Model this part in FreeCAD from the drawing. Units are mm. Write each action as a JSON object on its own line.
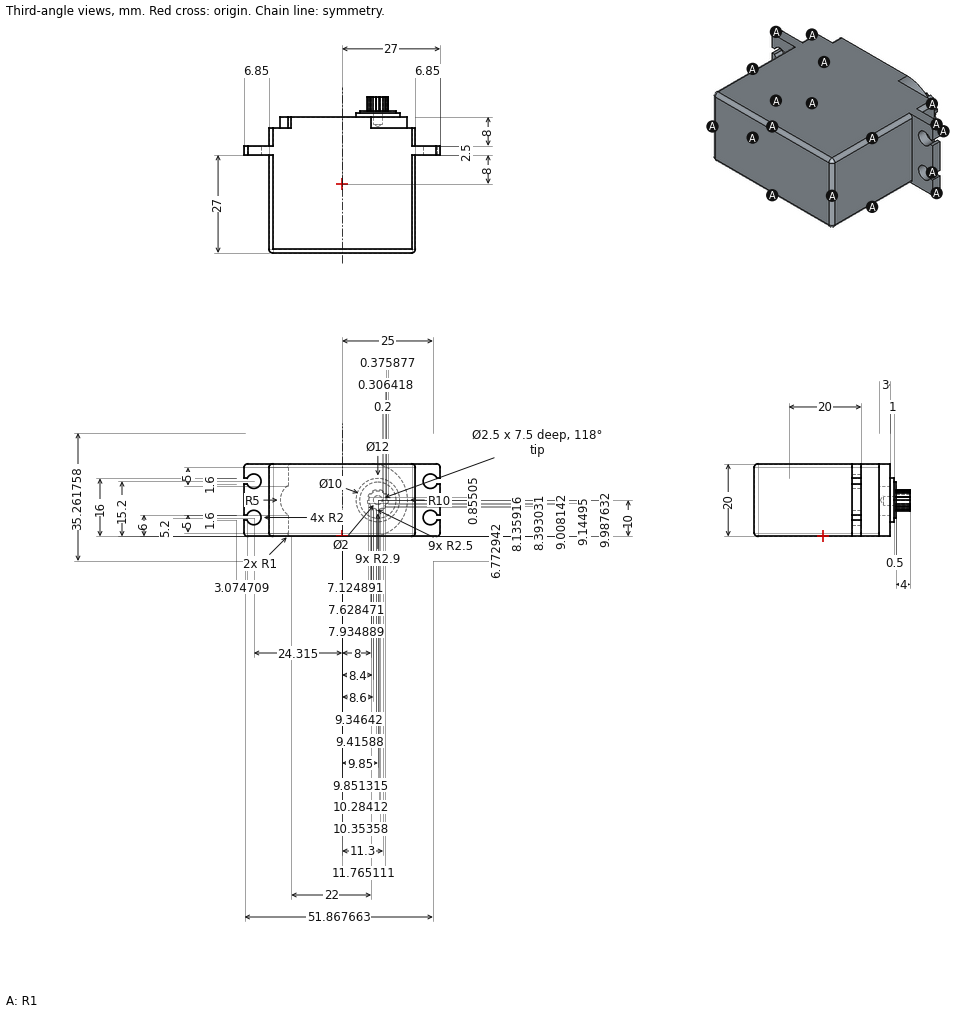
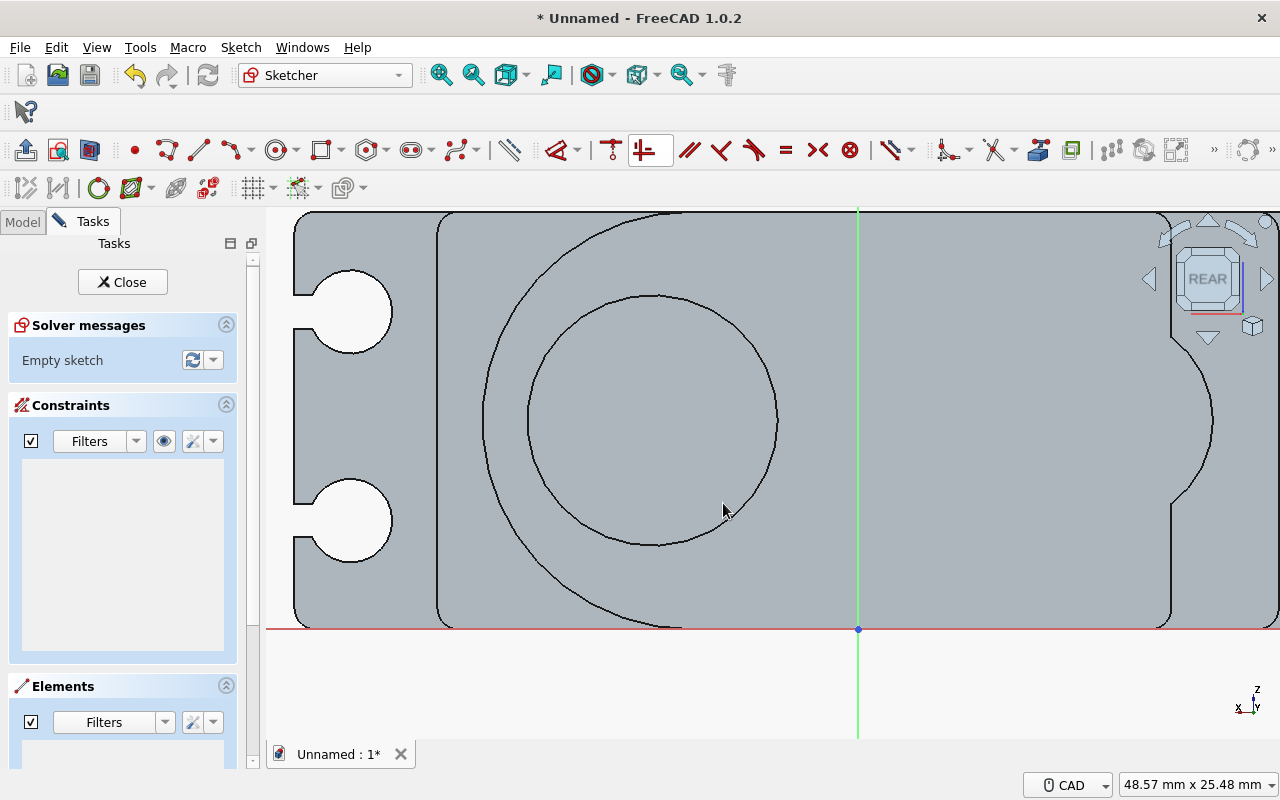
{"action": "left_click", "coordinate": [276, 150]}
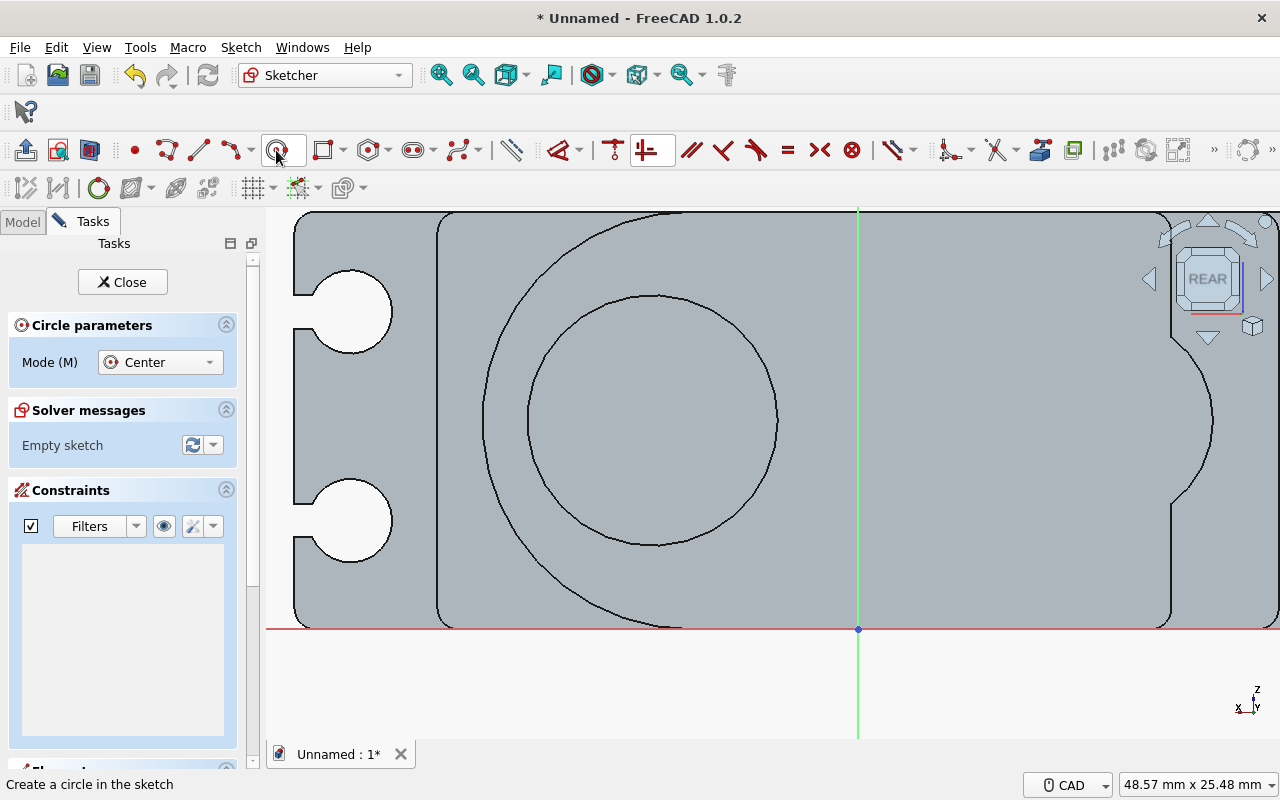
{"action": "left_click", "coordinate": [652, 421]}
{"action": "mouse_move", "coordinate": [726, 347]}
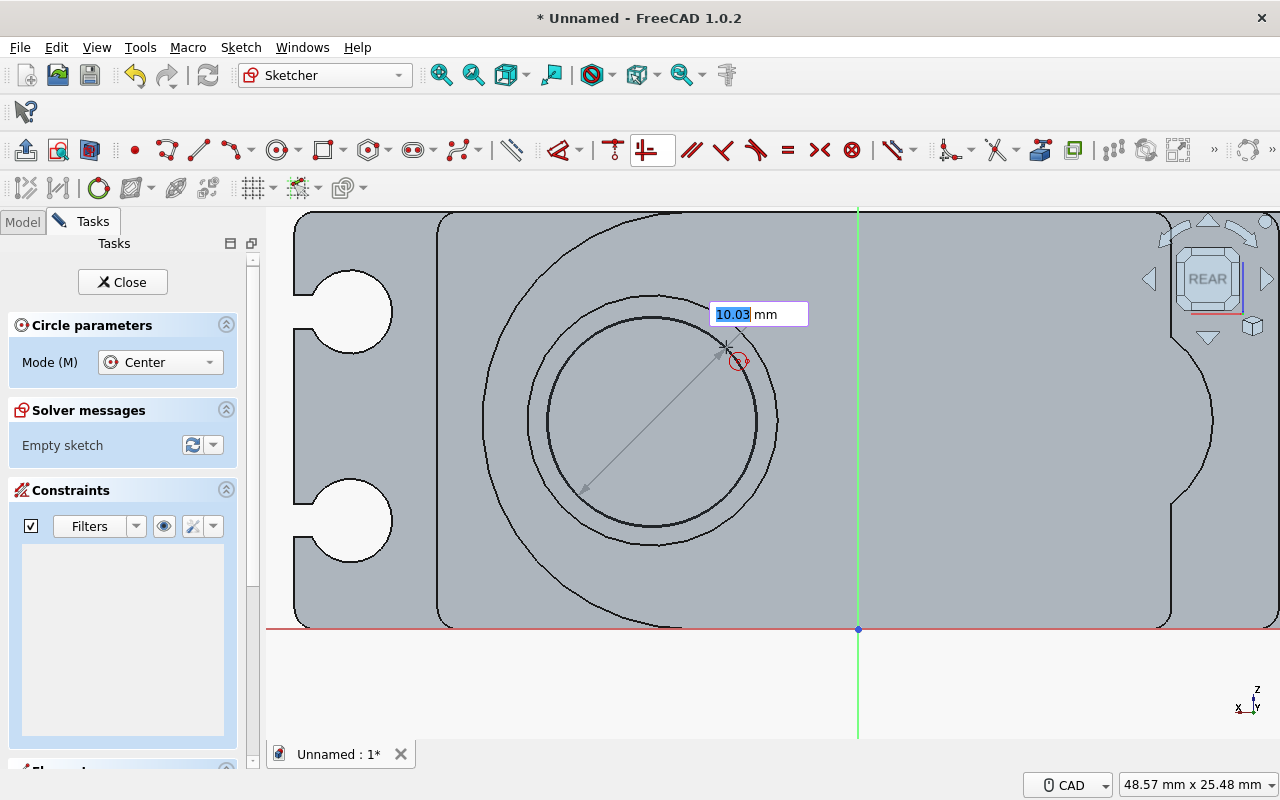
{"action": "type", "text": "10"}
{"action": "key", "text": "Return"}
{"action": "key", "text": "Escape"}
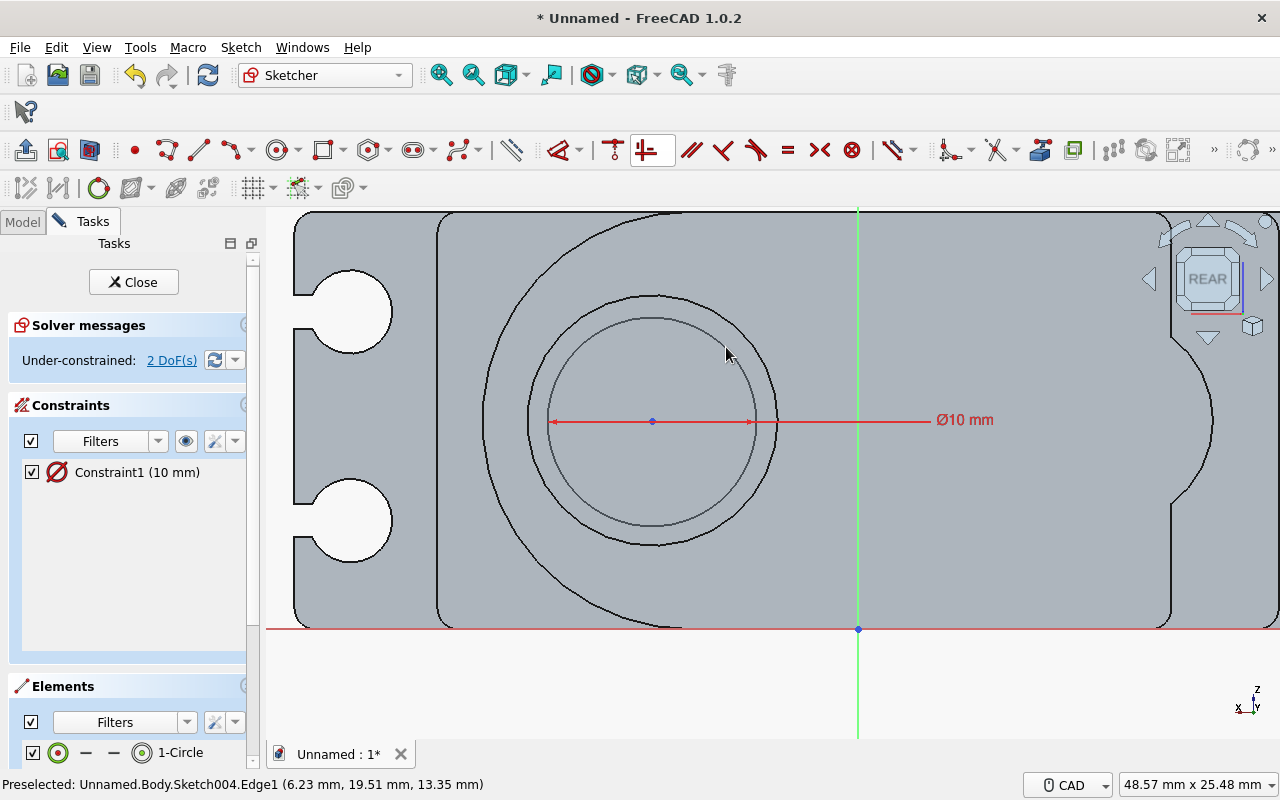
{"action": "left_click", "coordinate": [558, 150]}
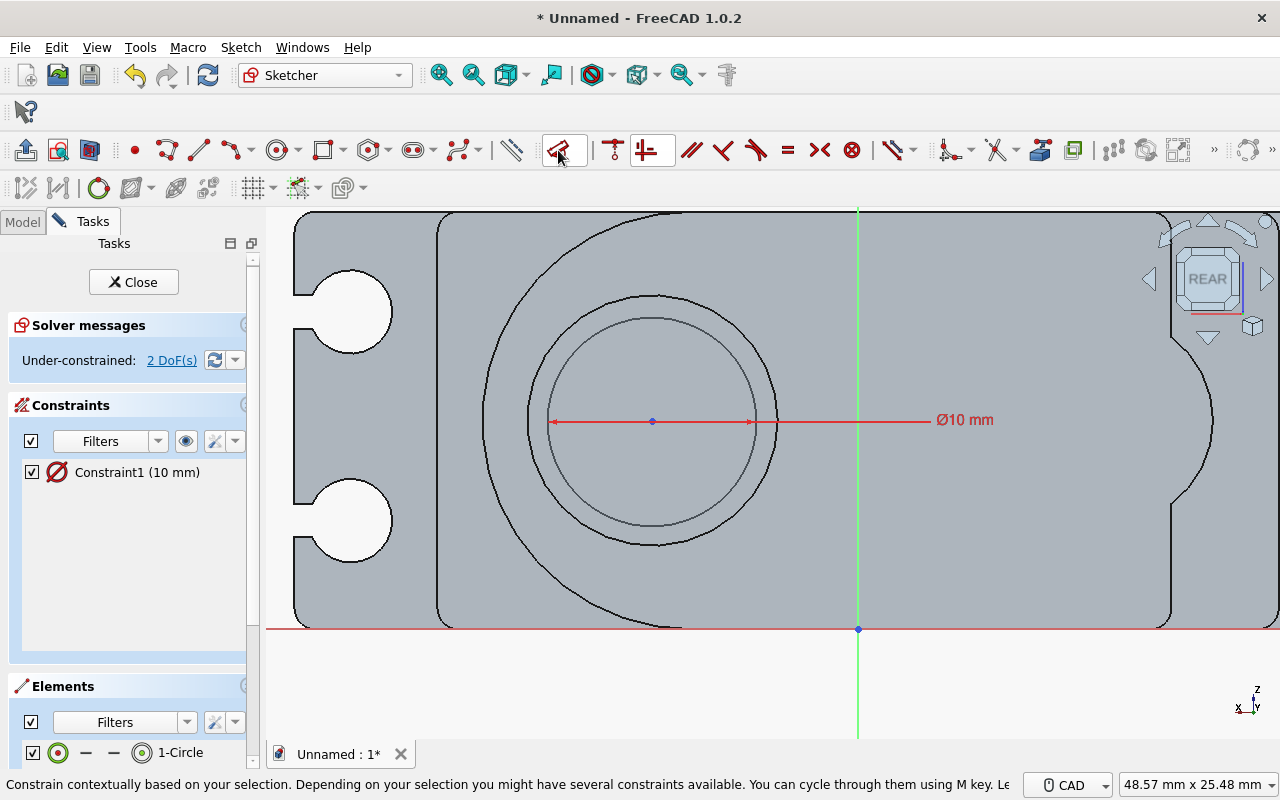
{"action": "left_click", "coordinate": [652, 422]}
{"action": "left_click", "coordinate": [755, 663]}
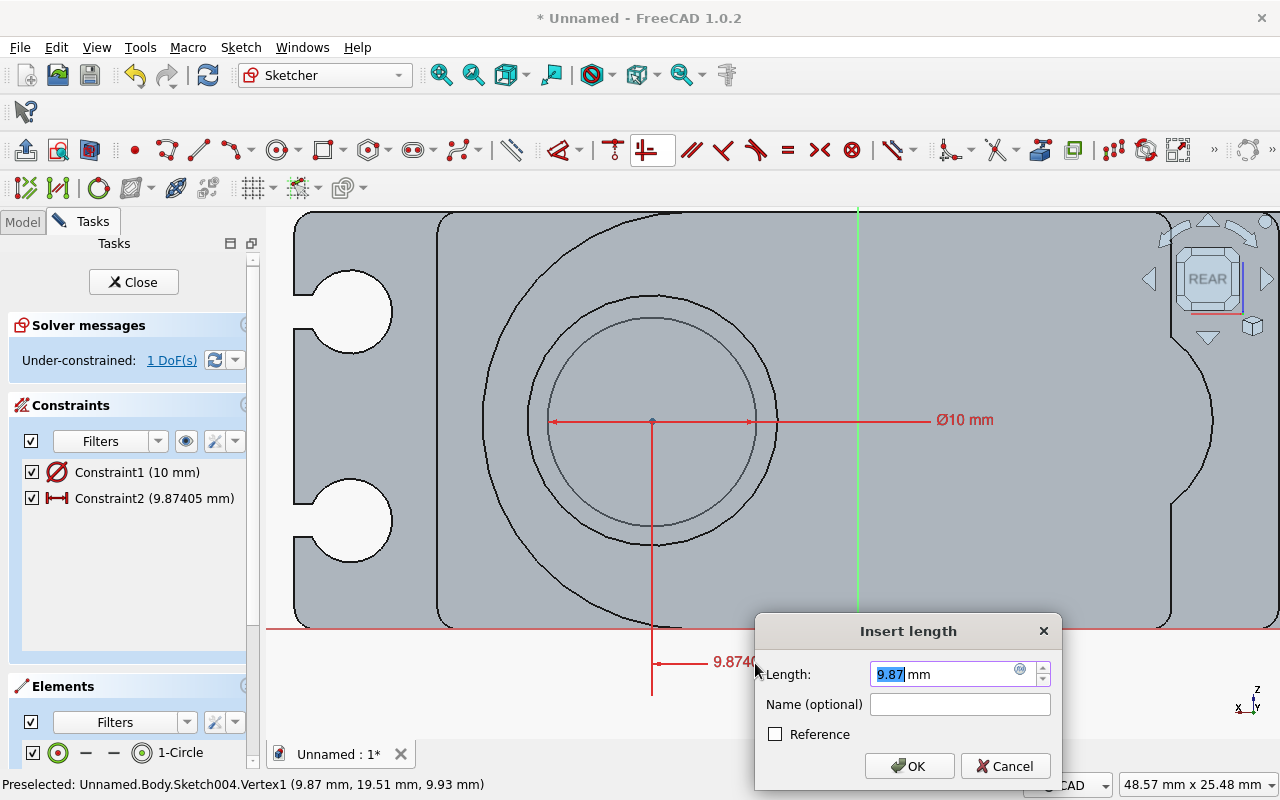
{"action": "type", "text": "9.851315"}
{"action": "key", "text": "Return"}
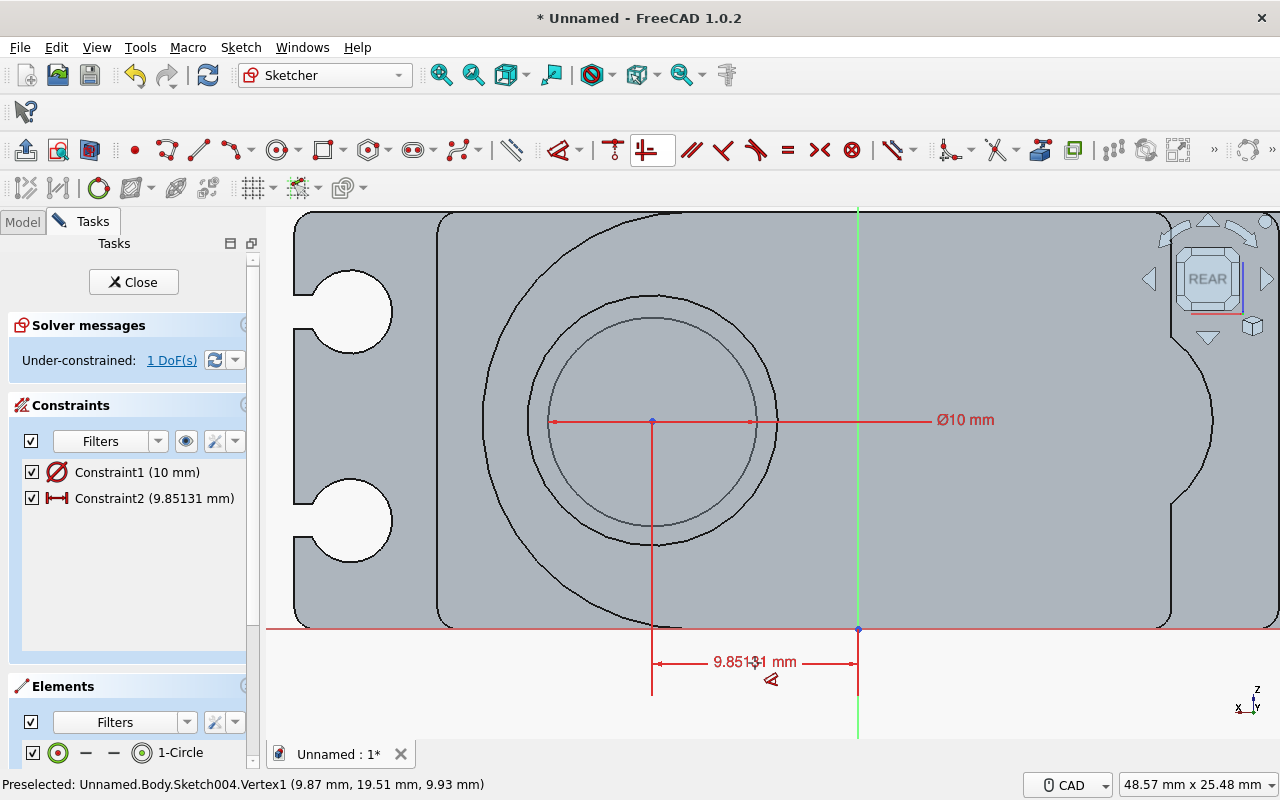
{"action": "left_click", "coordinate": [652, 422]}
{"action": "left_click", "coordinate": [892, 526]}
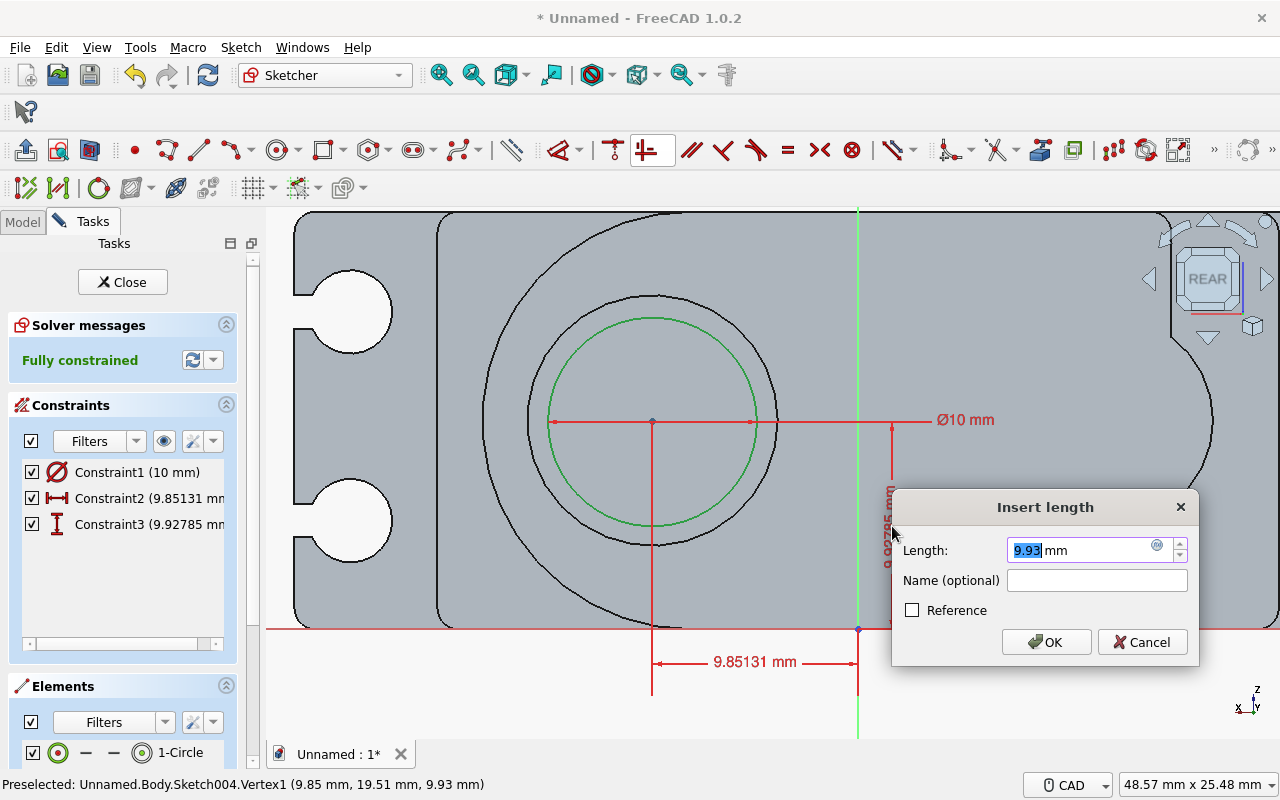
{"action": "type", "text": "9.987632"}
{"action": "key", "text": "Return"}
{"action": "key", "text": "Escape"}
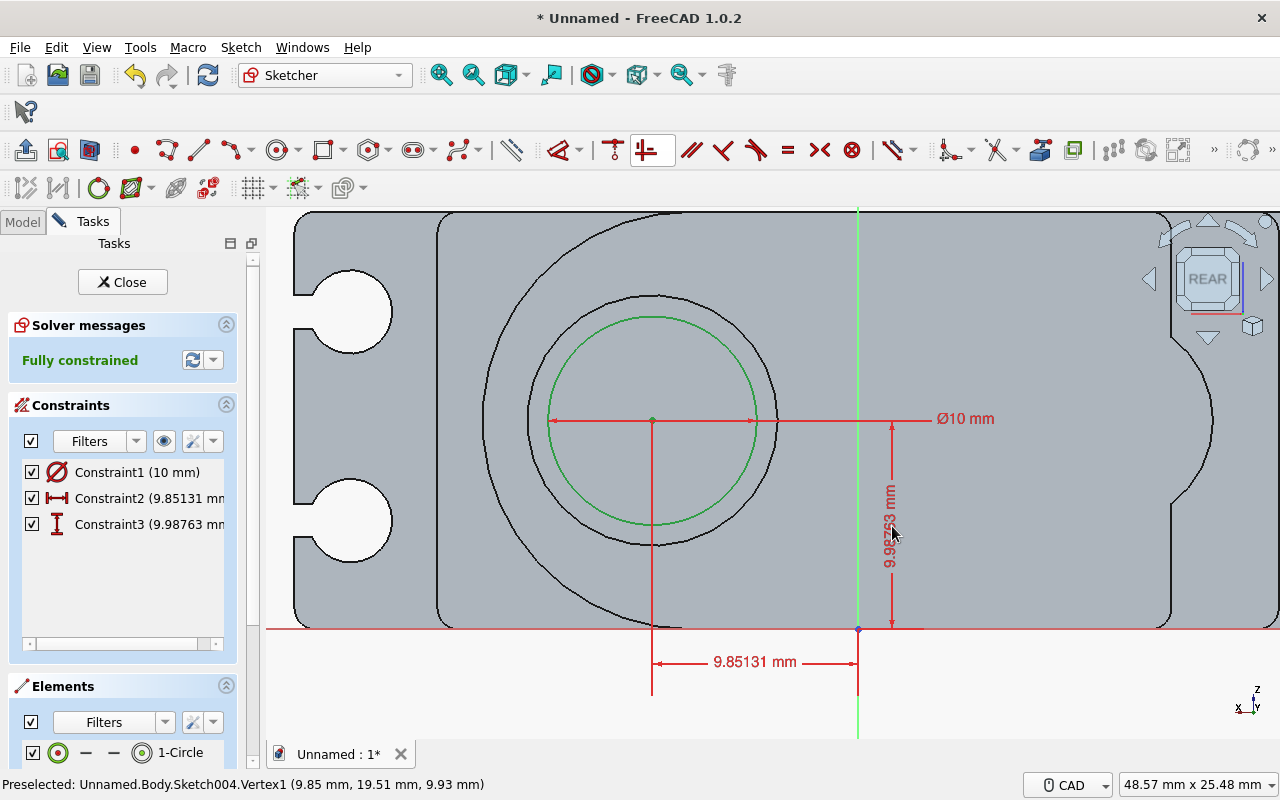
{"action": "left_click", "coordinate": [123, 282]}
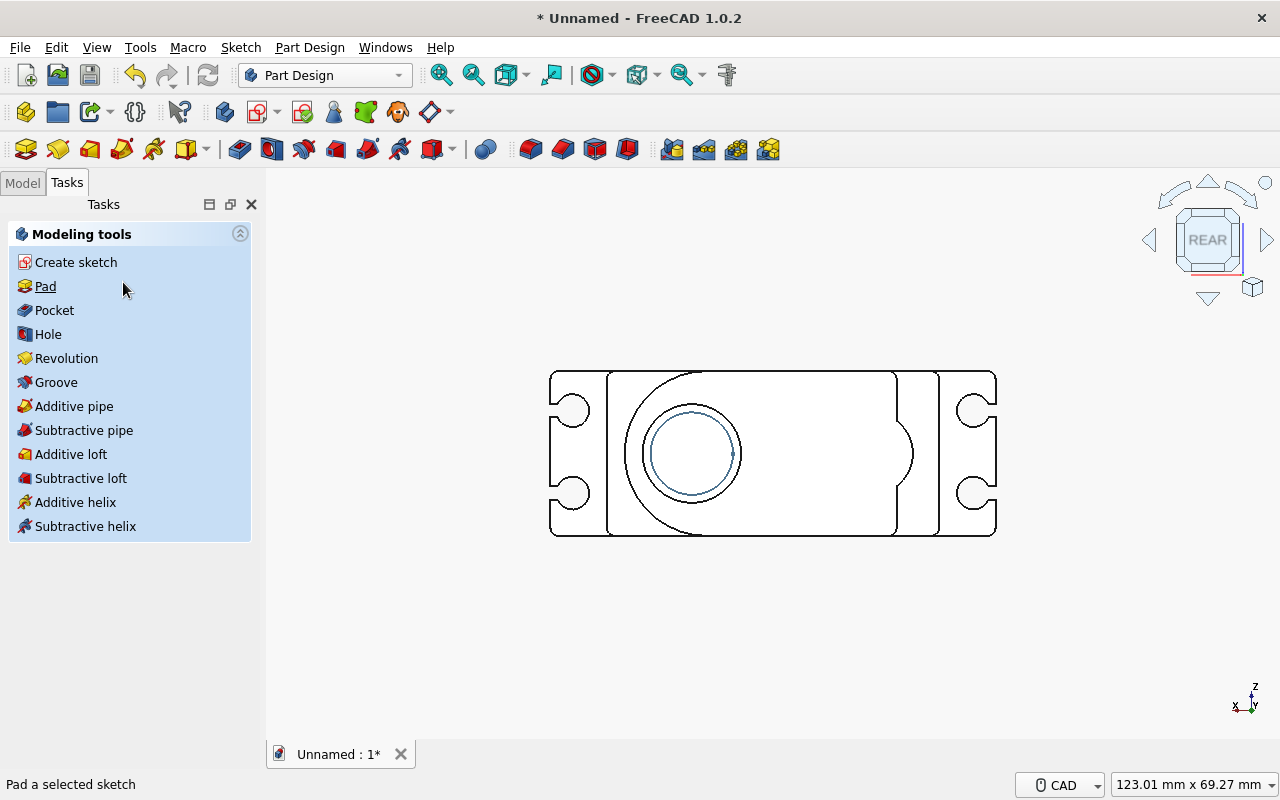
{"action": "left_click", "coordinate": [26, 150]}